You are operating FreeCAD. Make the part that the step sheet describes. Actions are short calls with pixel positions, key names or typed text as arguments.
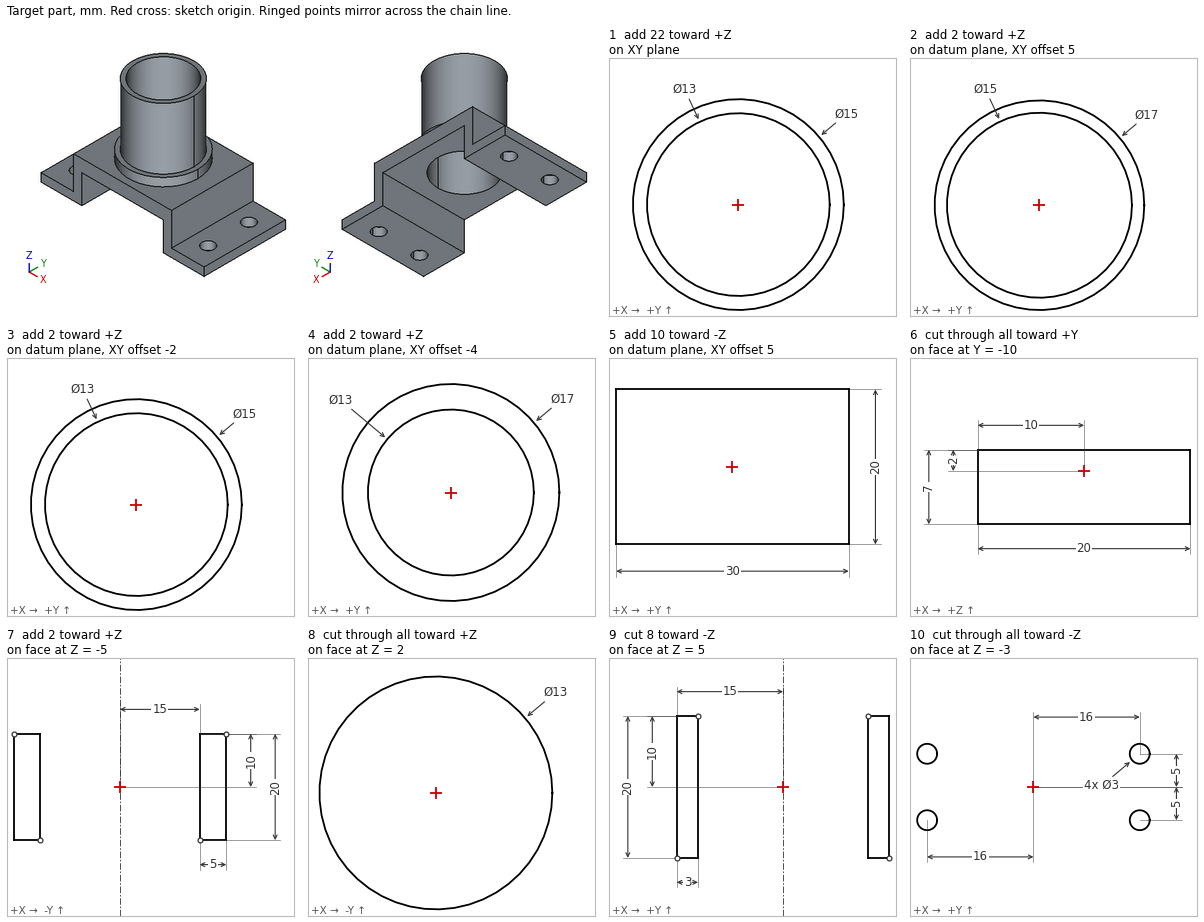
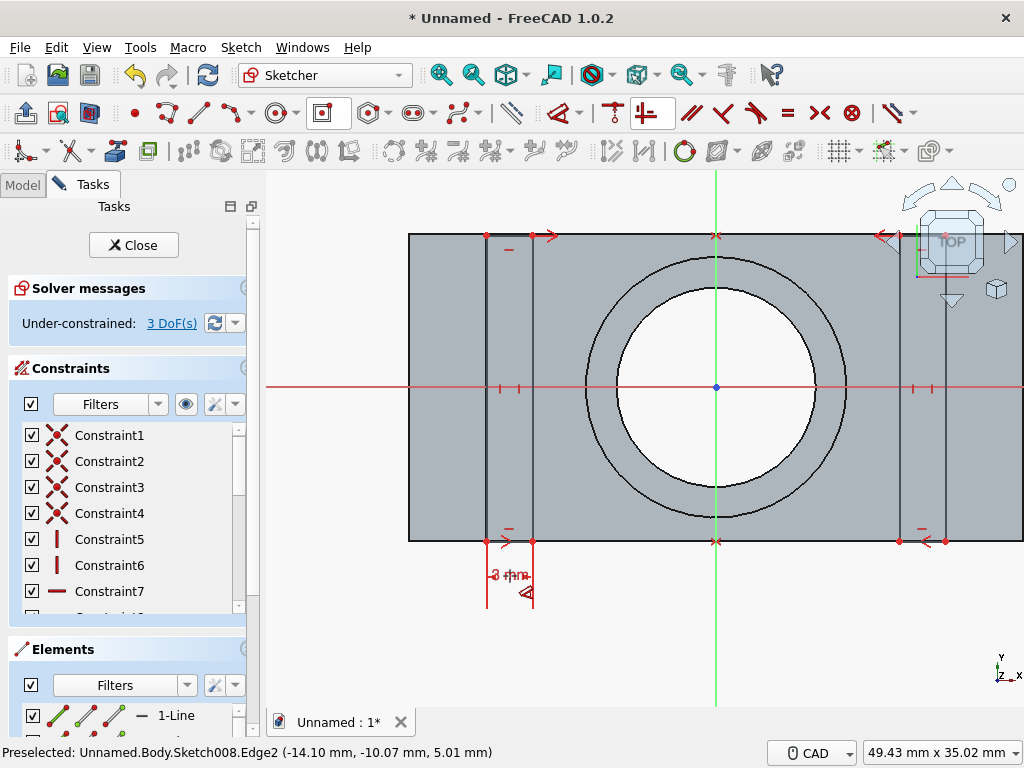
click(487, 328)
click(453, 318)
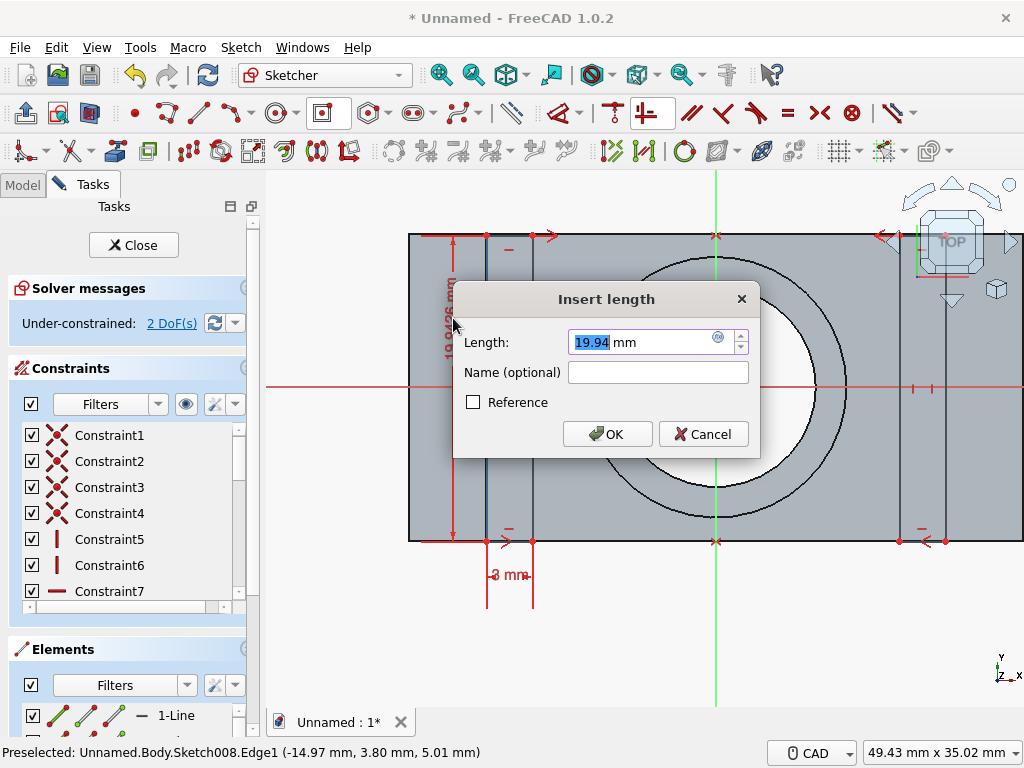
text(20)
key(Return)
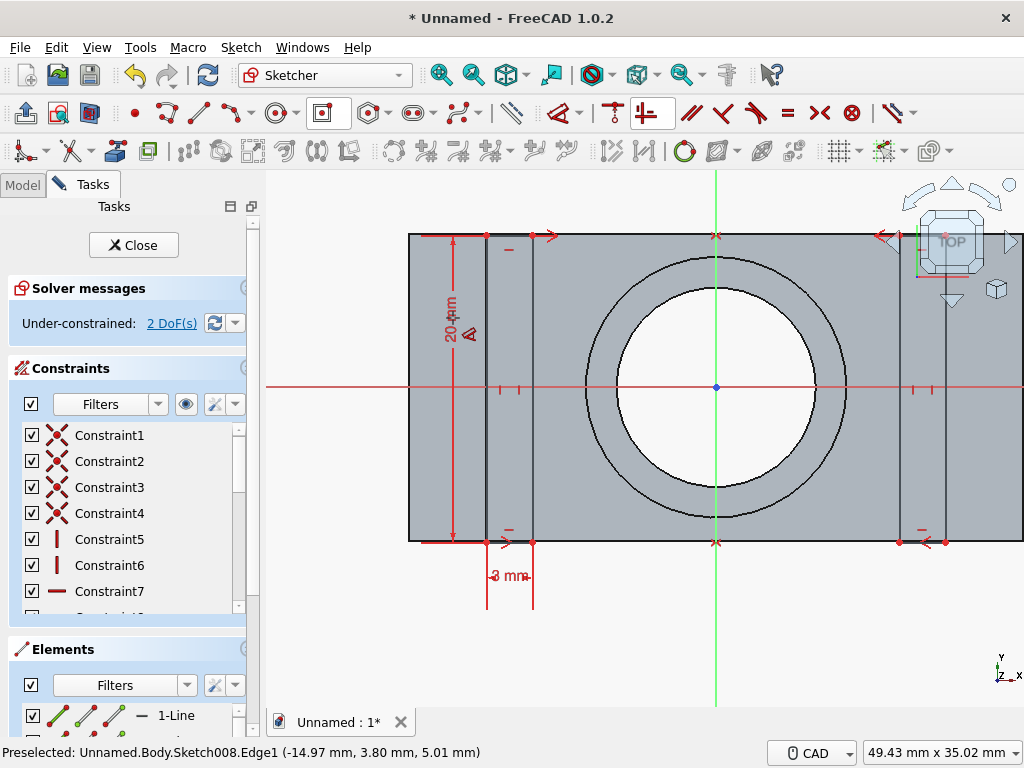
click(487, 236)
click(601, 202)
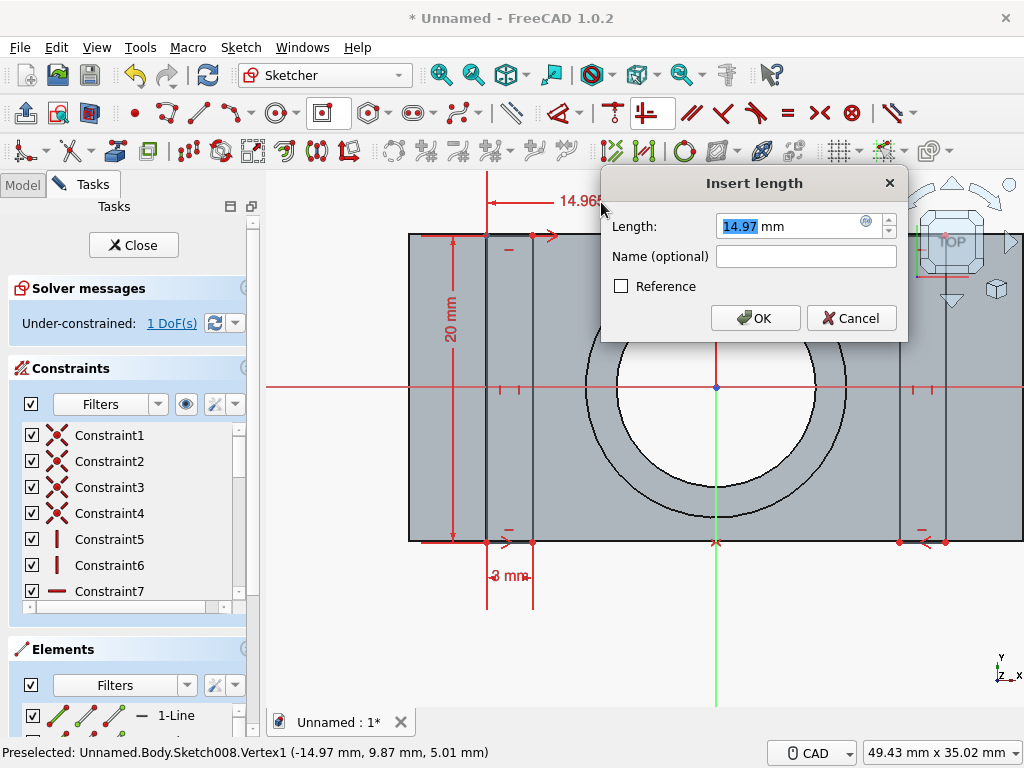
text(15)
key(Return)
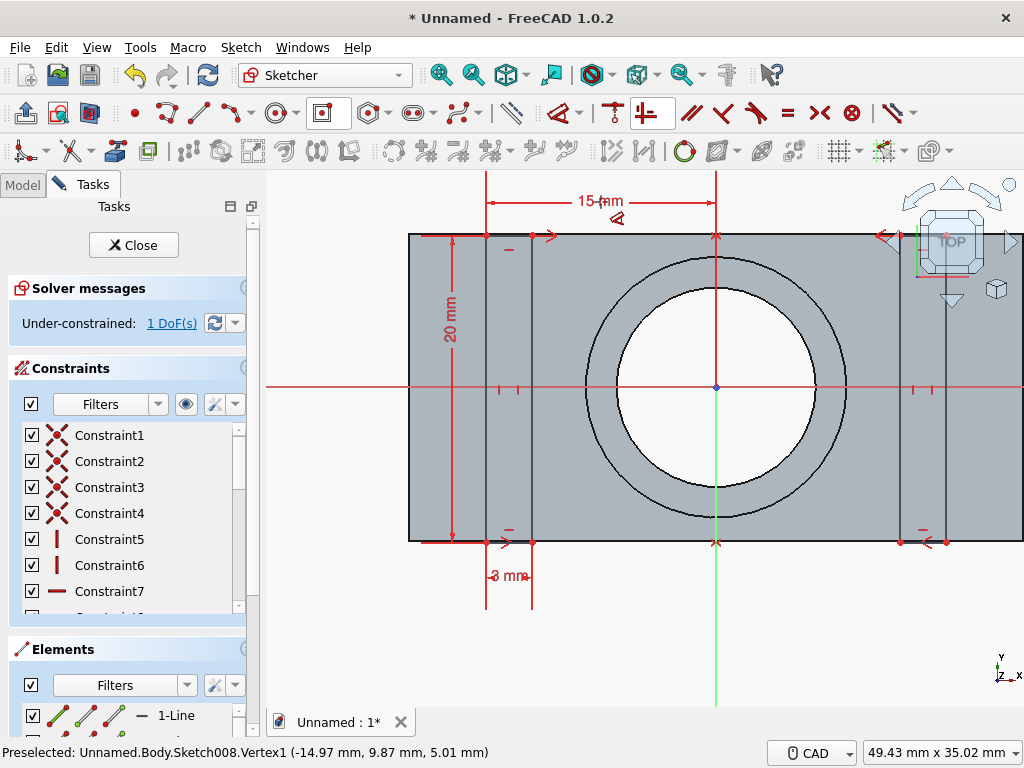
click(486, 236)
click(452, 277)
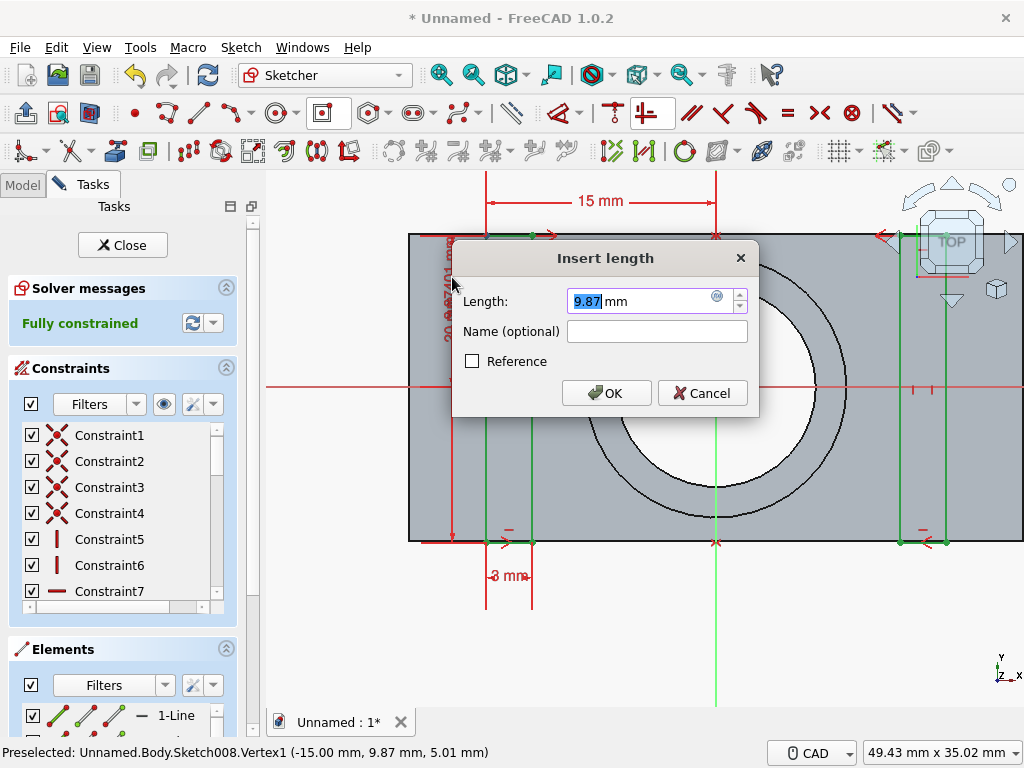
text(10)
key(Return)
key(Escape)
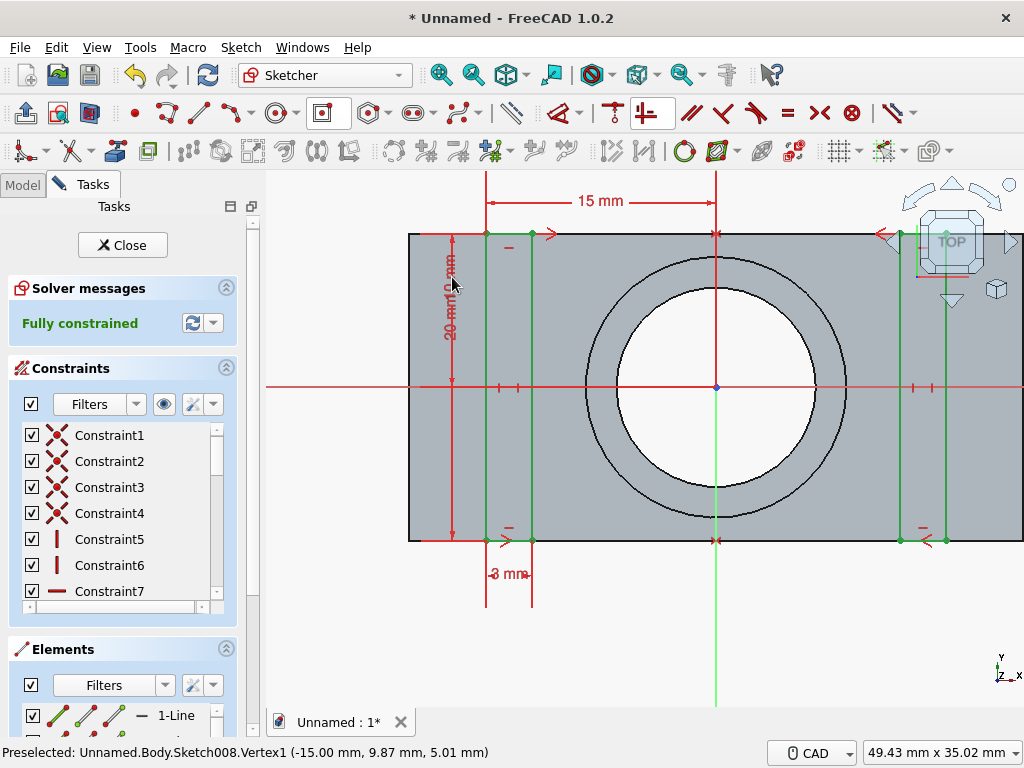
click(123, 245)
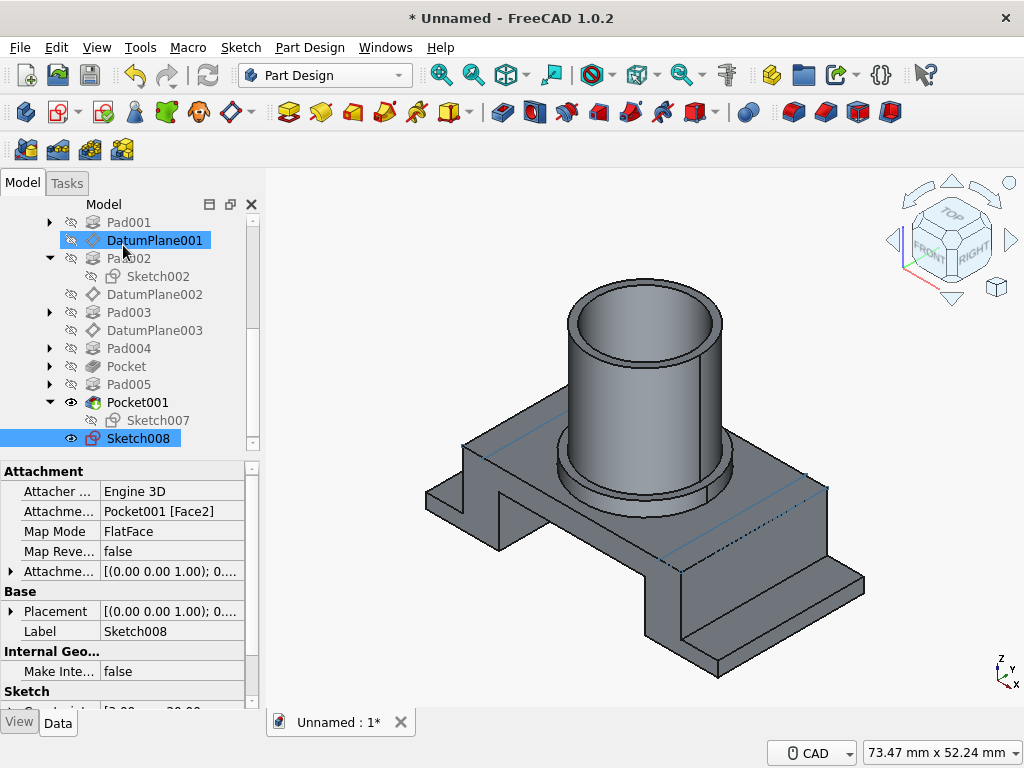
click(504, 112)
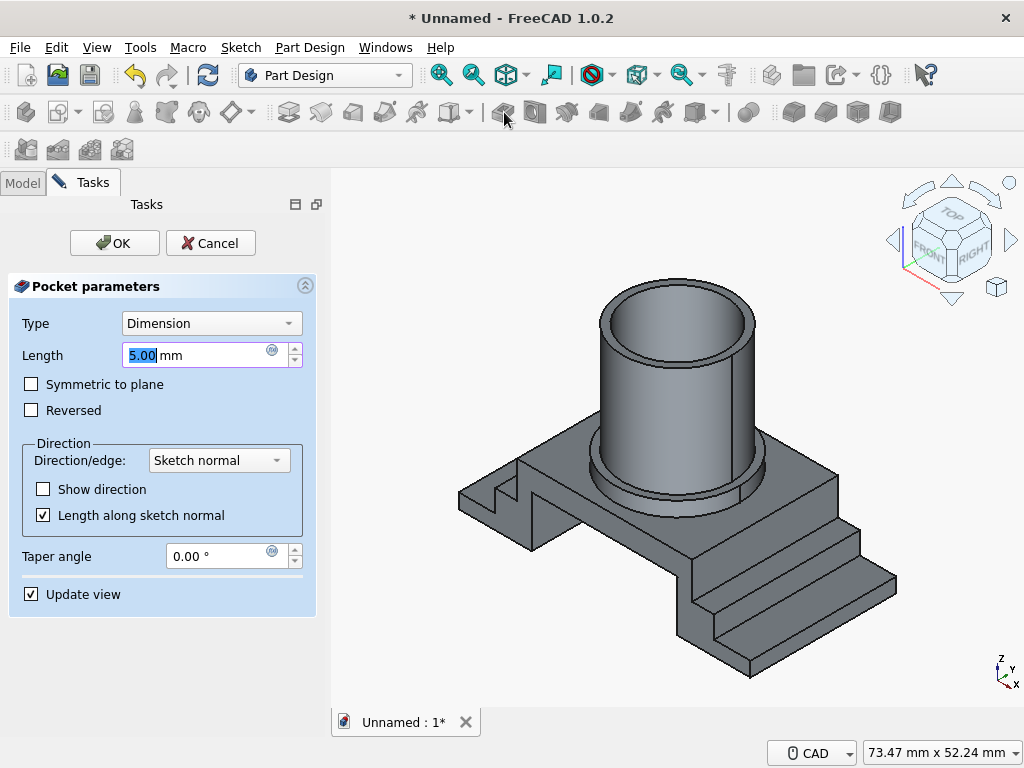
text(8)
key(Tab)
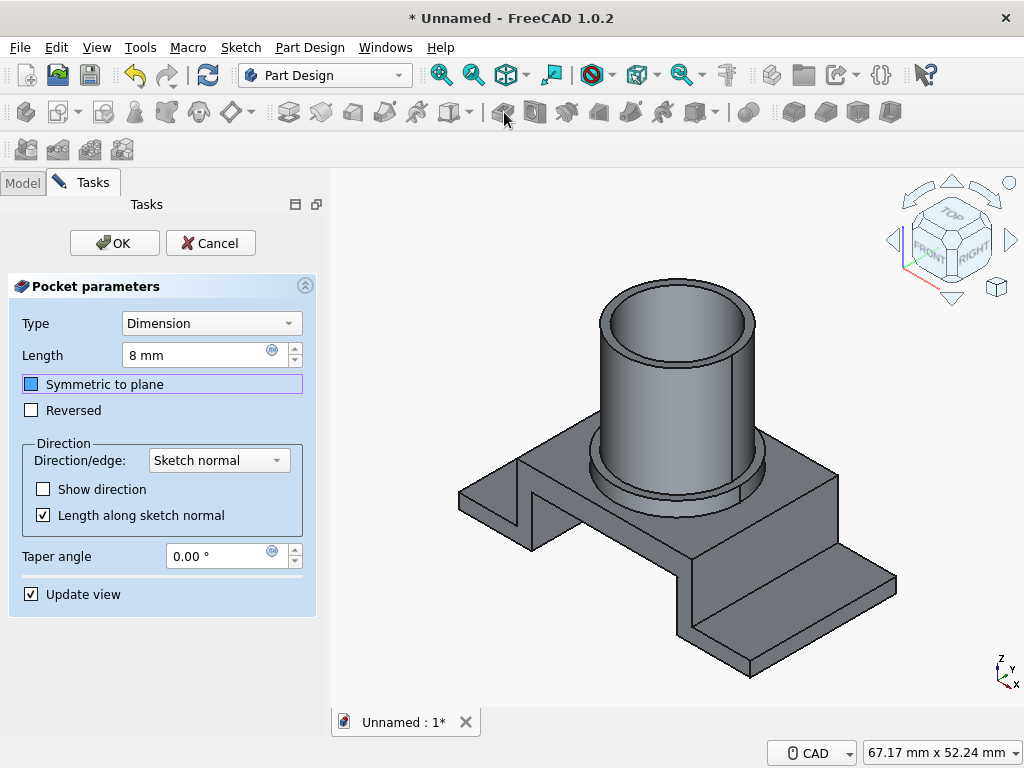
click(115, 243)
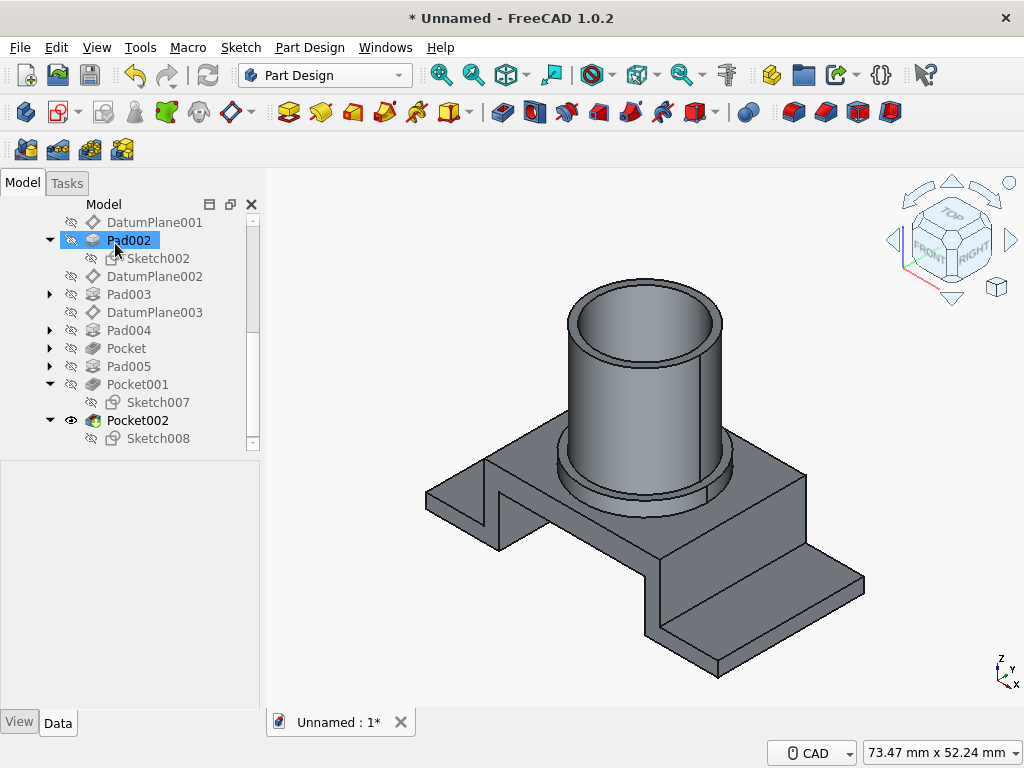
click(803, 577)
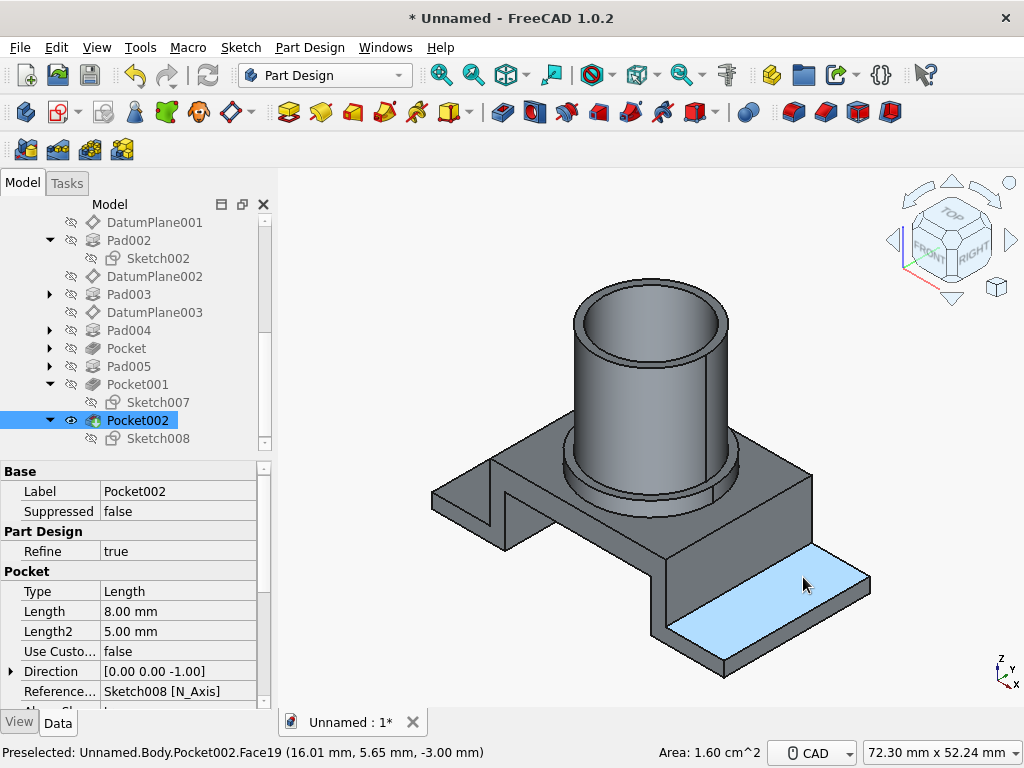
click(58, 112)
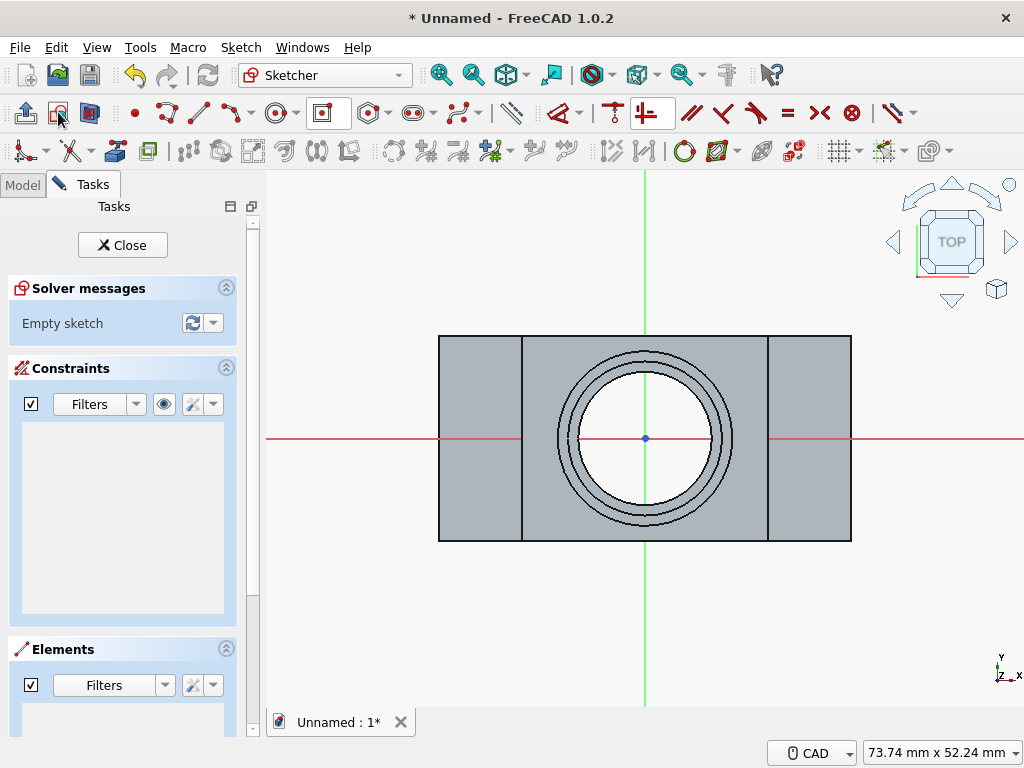
key(q)
key(s)